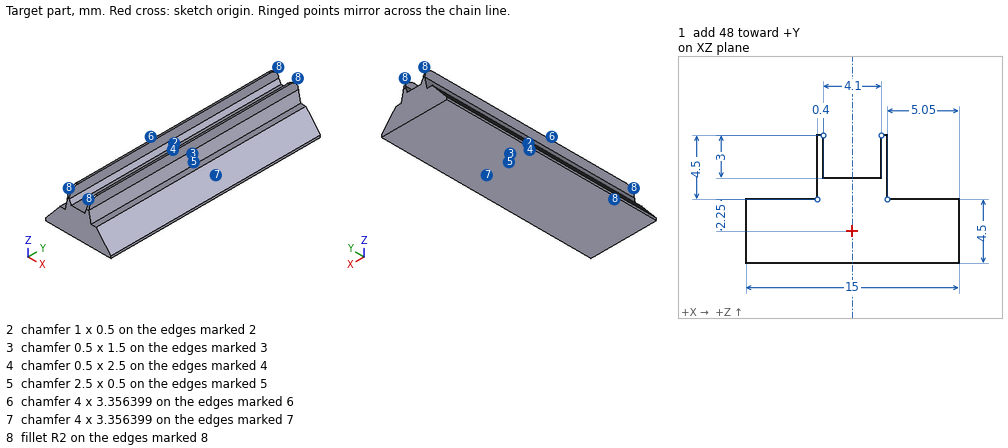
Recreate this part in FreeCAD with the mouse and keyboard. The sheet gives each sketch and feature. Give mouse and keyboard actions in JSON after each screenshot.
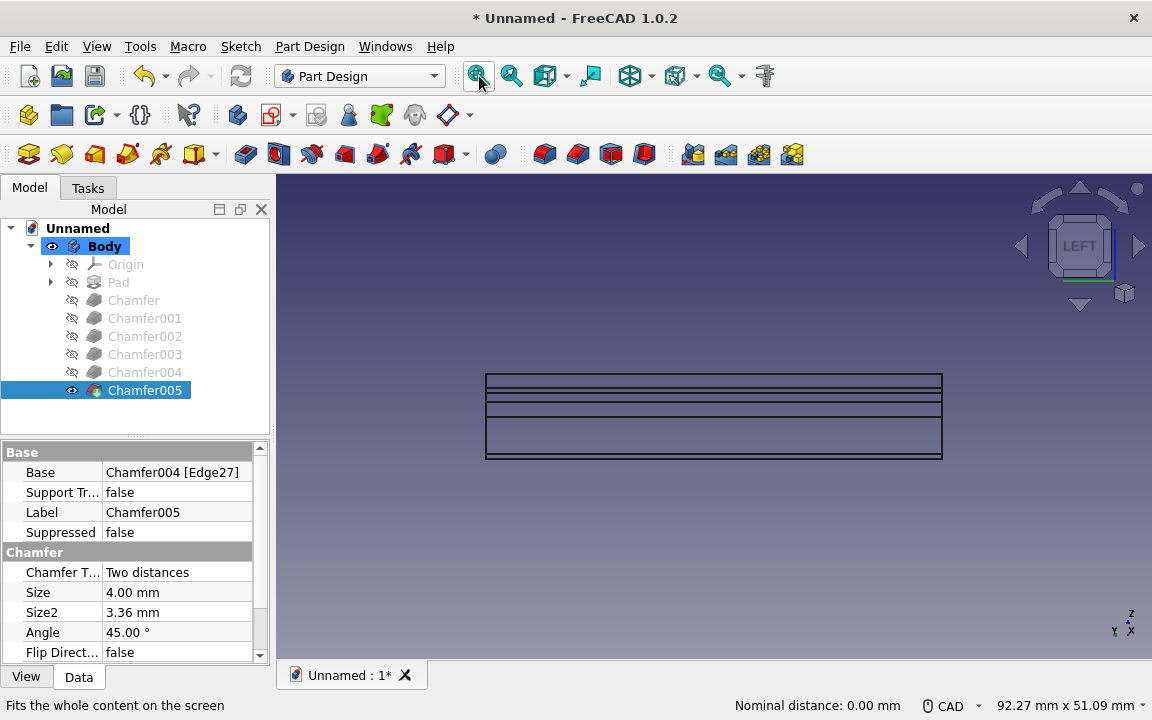
{"action": "key", "text": "0"}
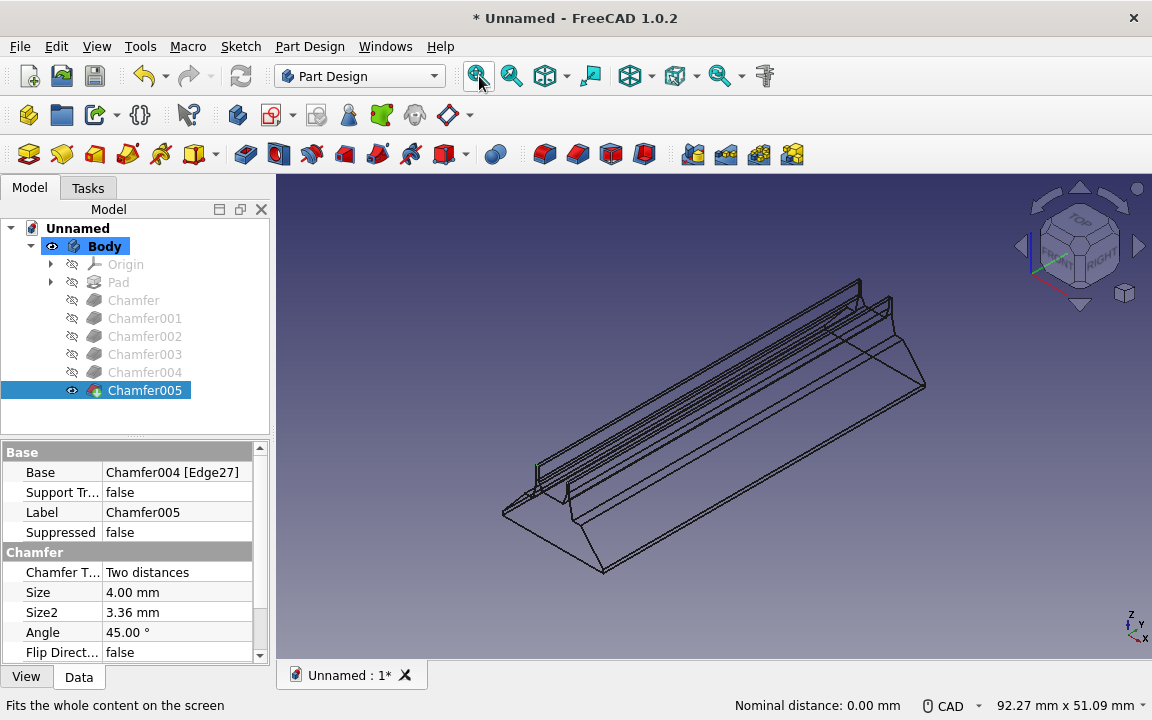
{"action": "scroll", "coordinate": [860, 279], "scroll_direction": "up", "scroll_amount": 12}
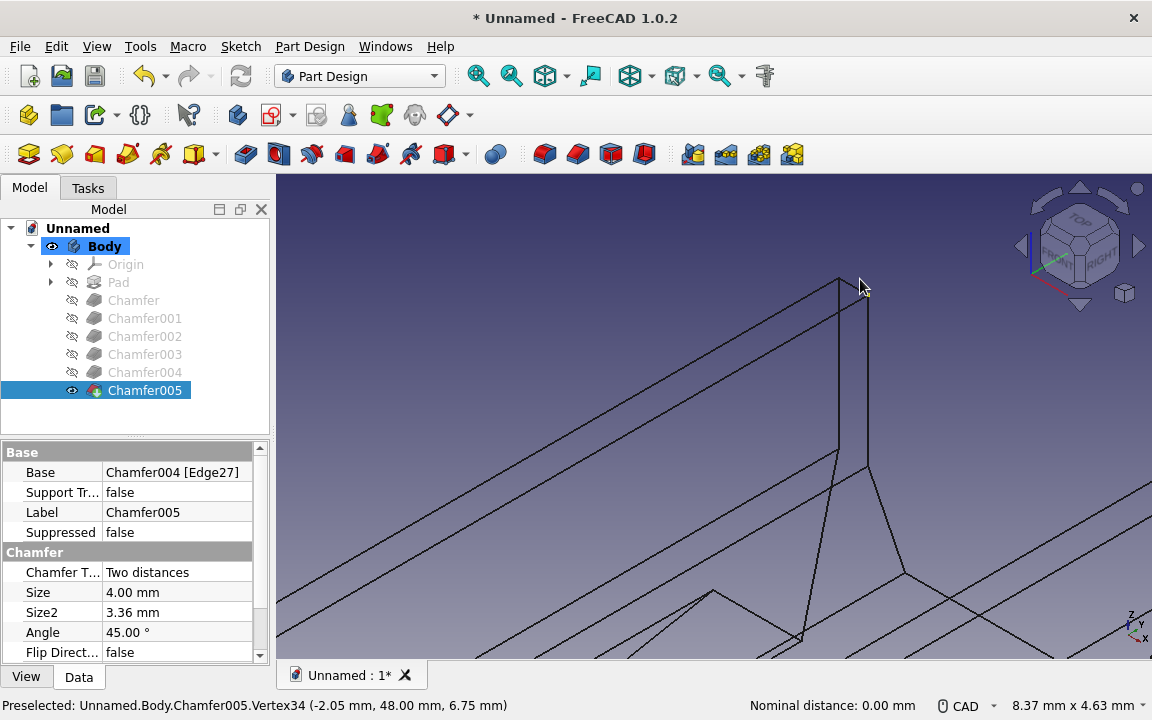
{"action": "left_click", "coordinate": [853, 286], "text": "ctrl"}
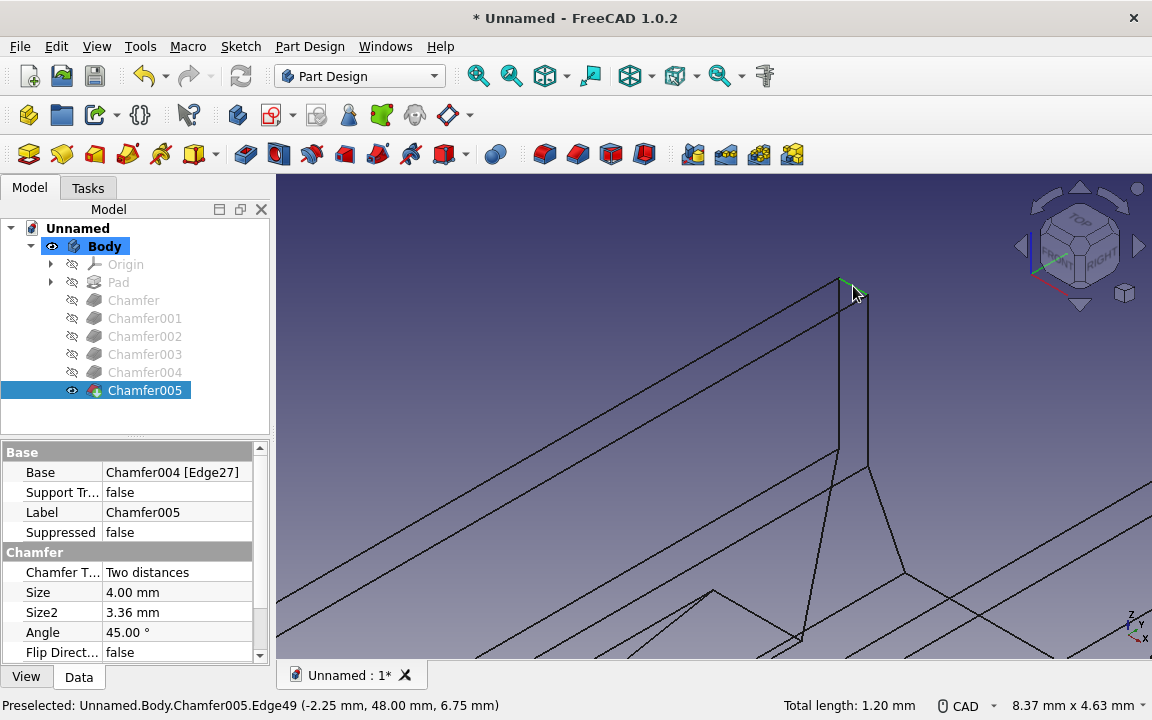
{"action": "key", "text": "v f"}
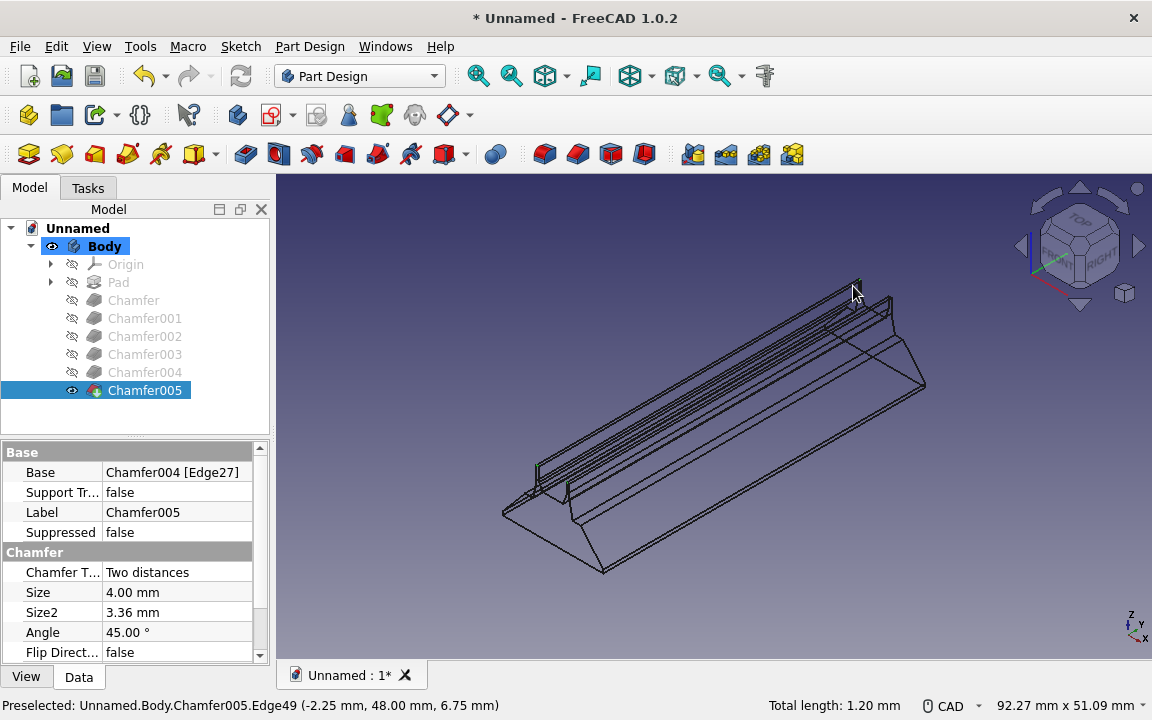
{"action": "key", "text": "2"}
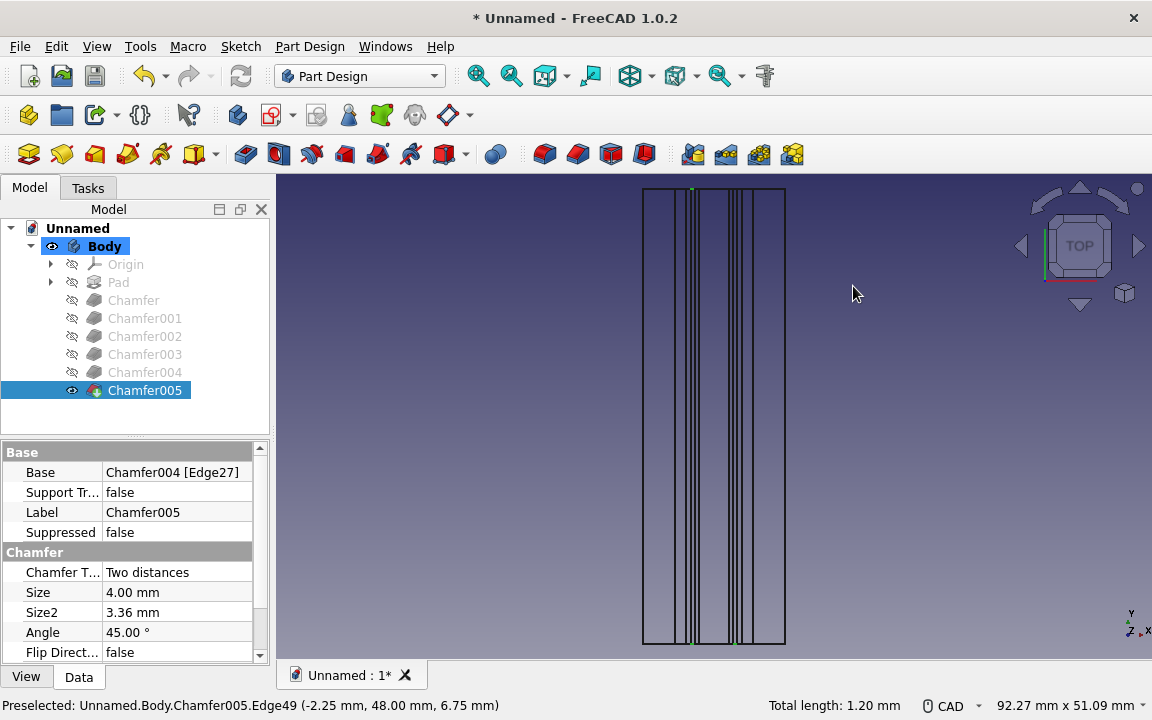
{"action": "key", "text": "1"}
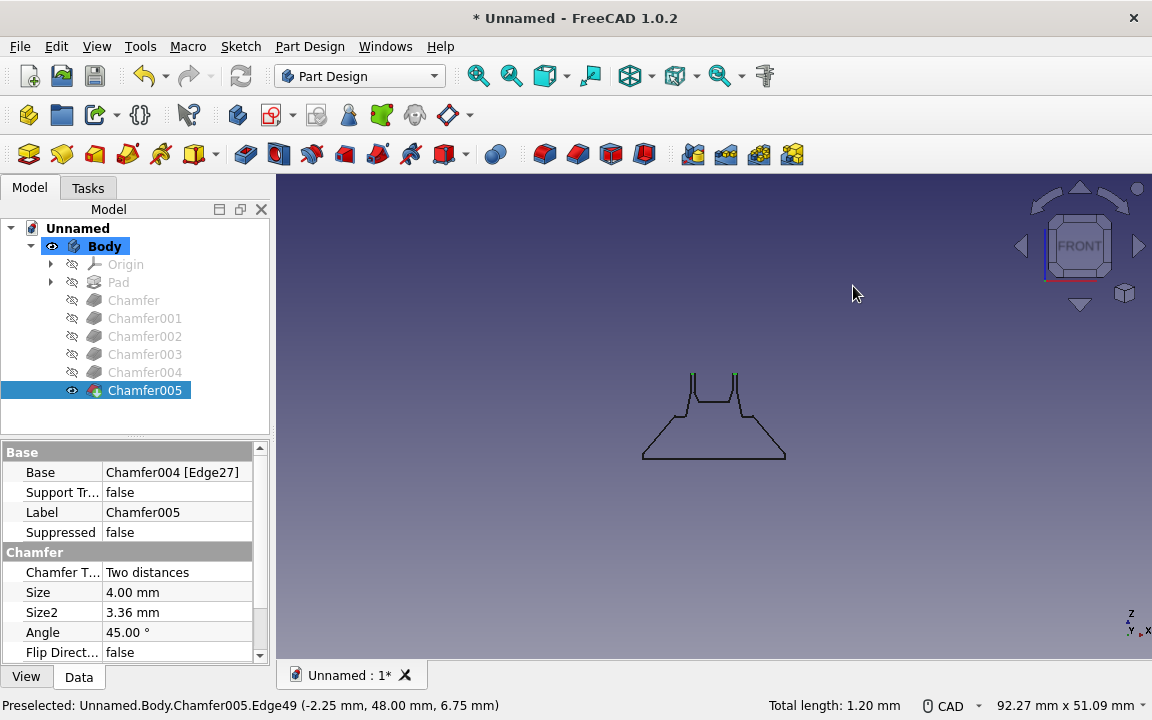
{"action": "left_click", "coordinate": [479, 76]}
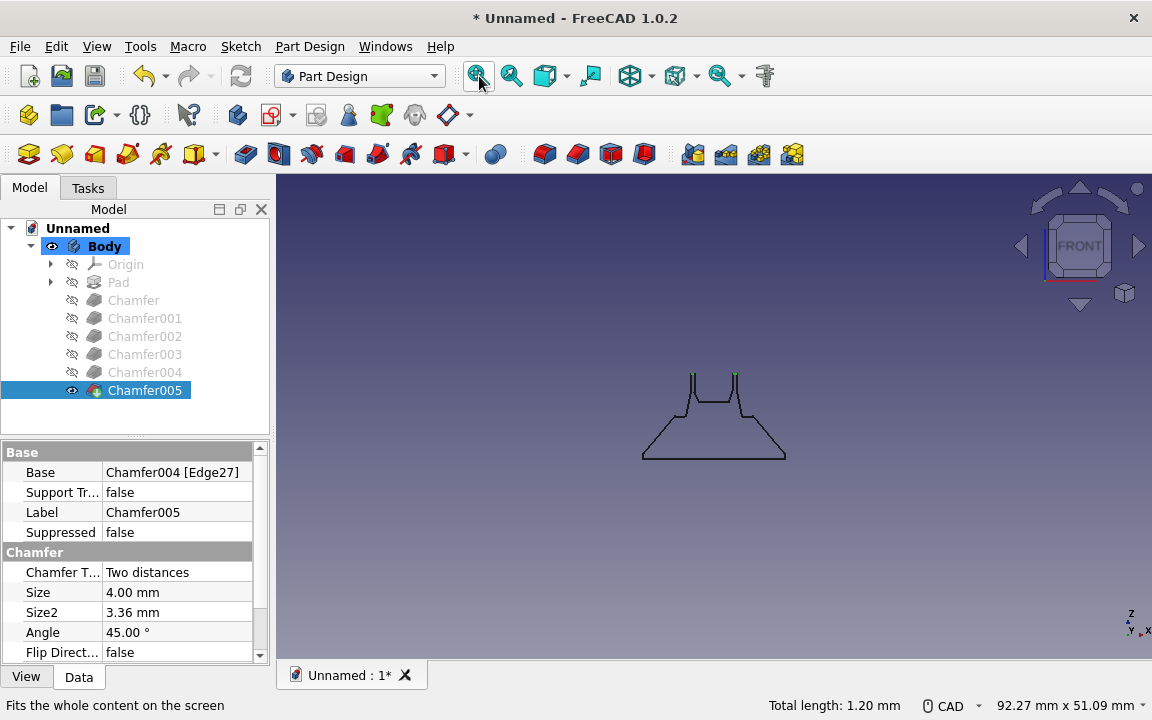
{"action": "scroll", "coordinate": [735, 373], "scroll_direction": "up", "scroll_amount": 12}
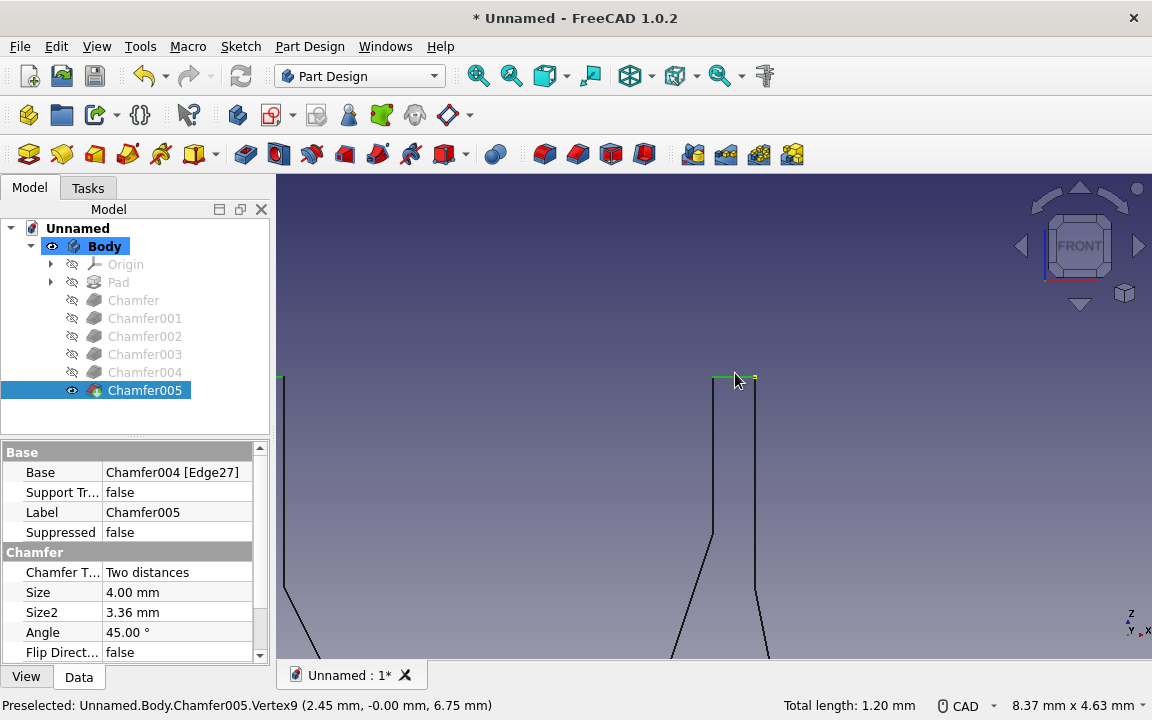
{"action": "key", "text": "v f"}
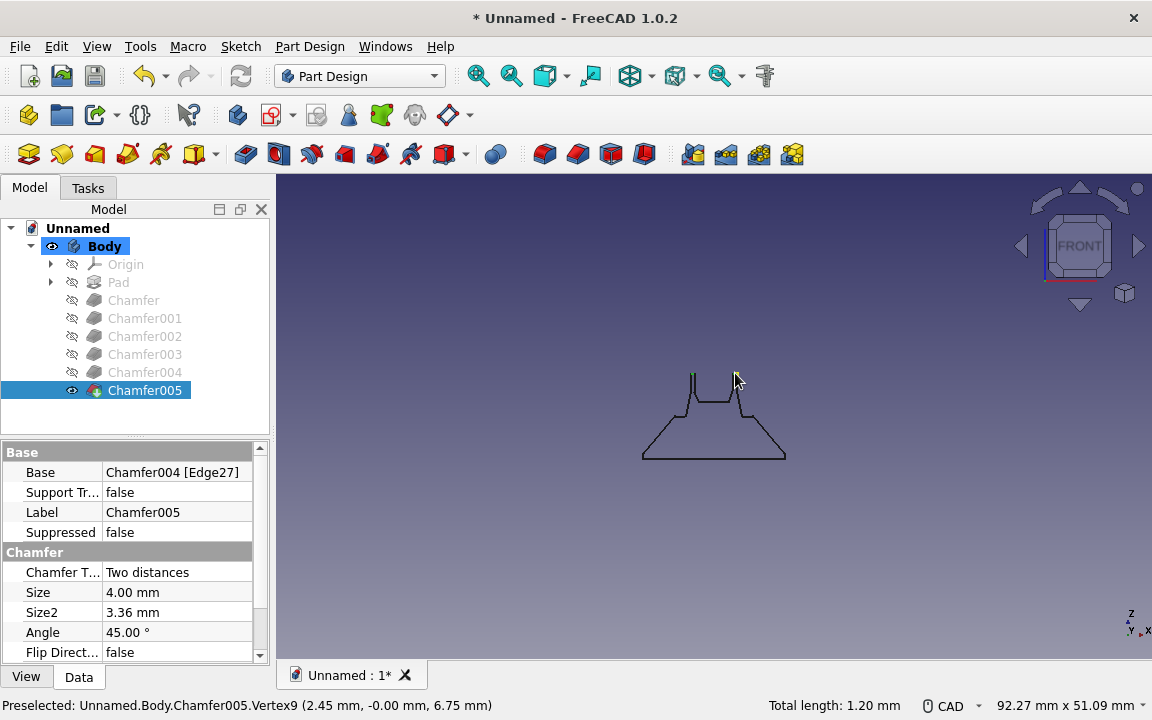
{"action": "key", "text": "3"}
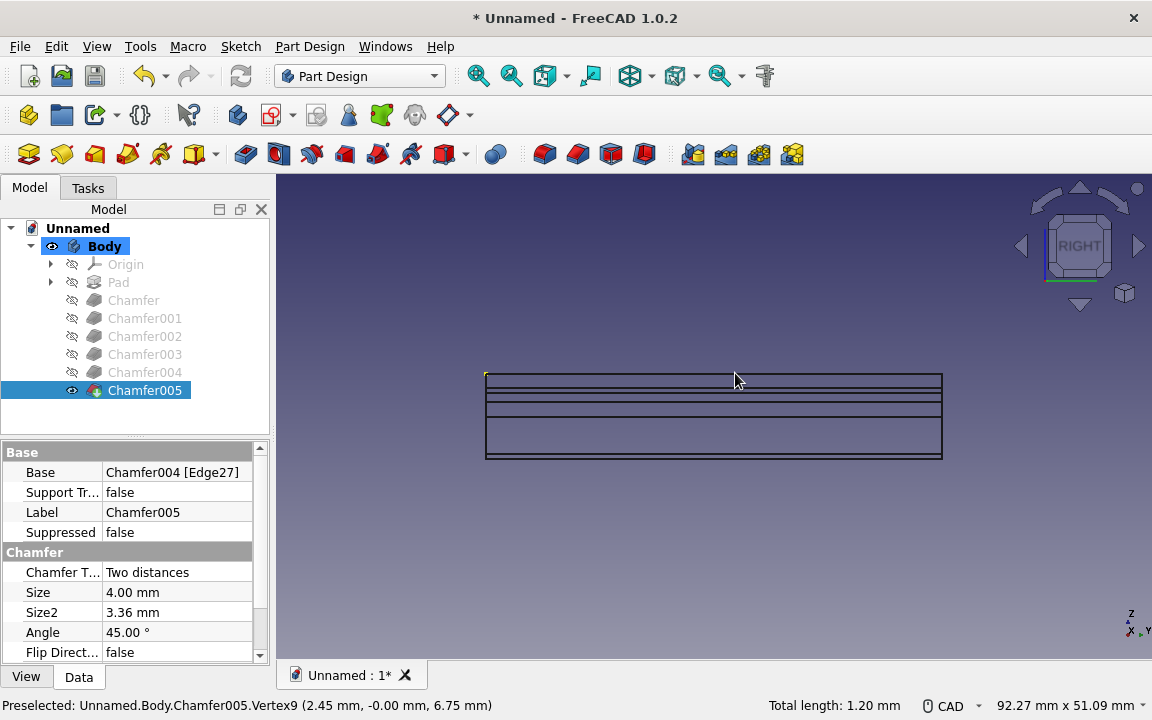
{"action": "scroll", "coordinate": [942, 373], "scroll_direction": "up", "scroll_amount": 12}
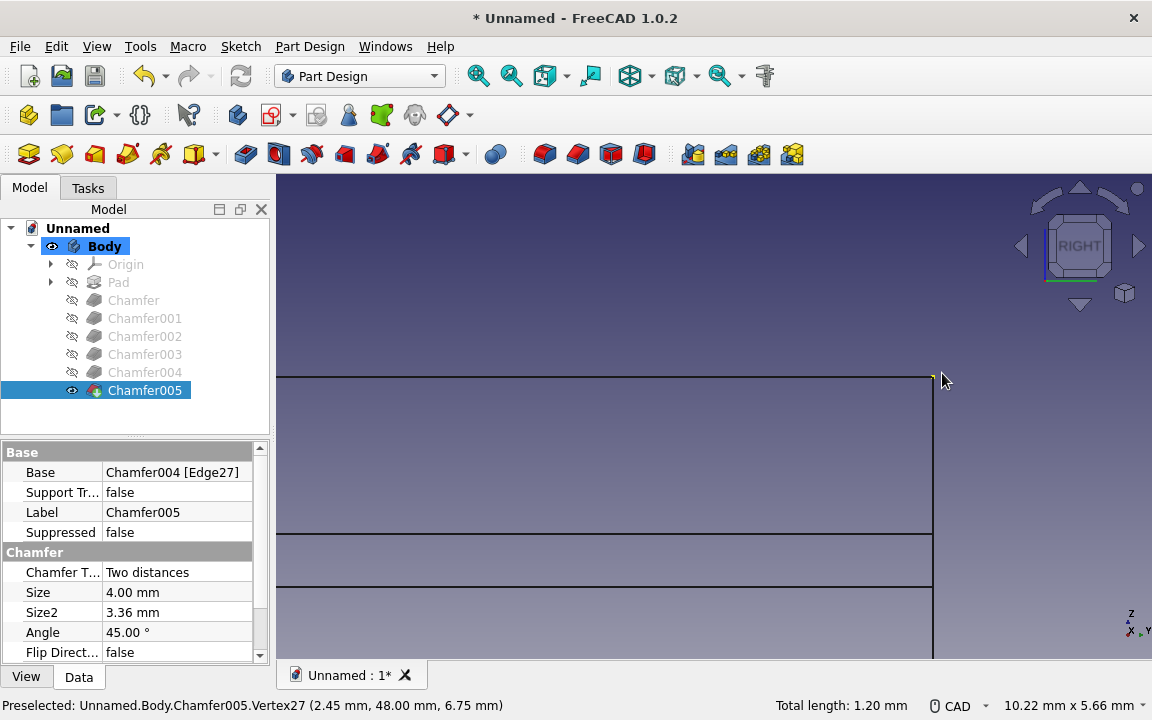
{"action": "key", "text": "v f"}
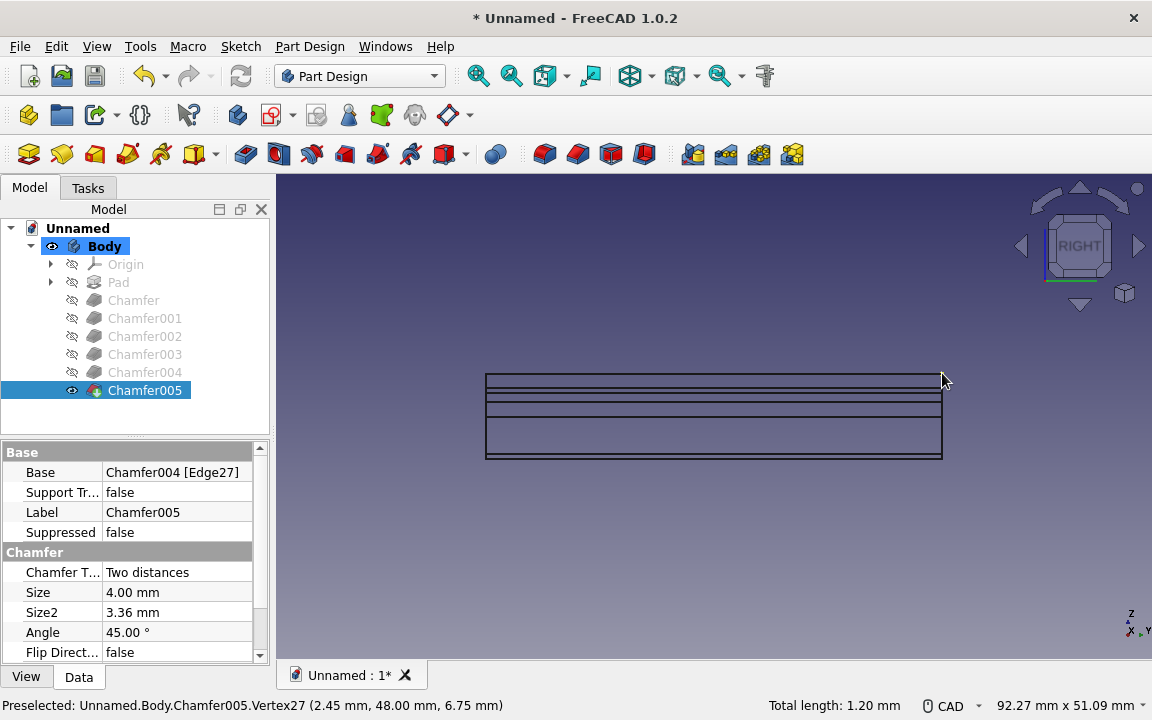
{"action": "key", "text": "5"}